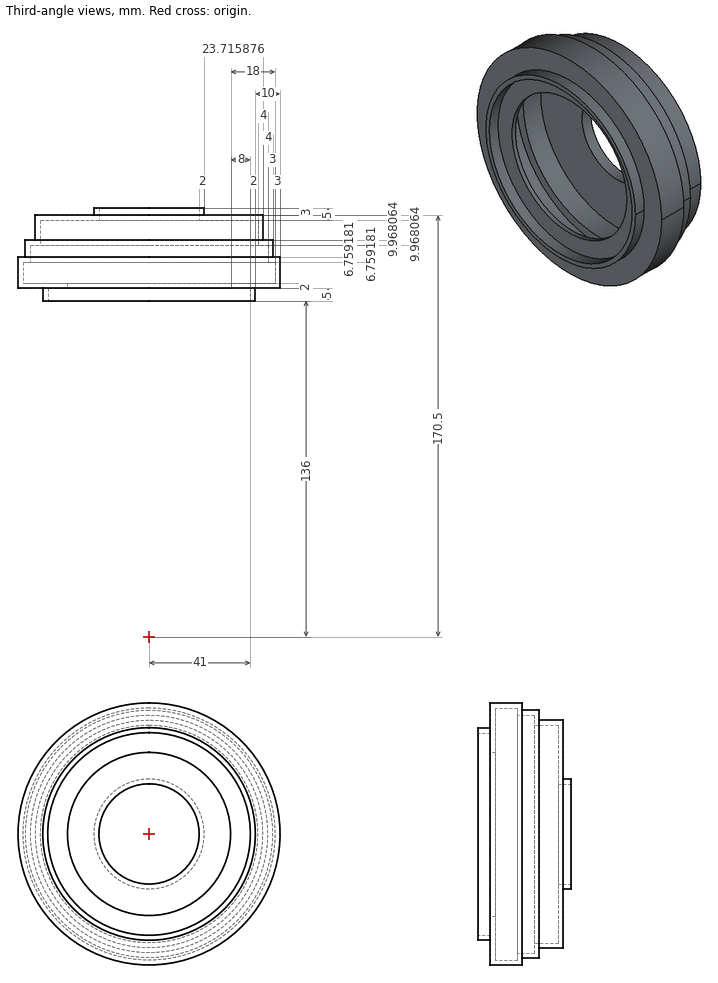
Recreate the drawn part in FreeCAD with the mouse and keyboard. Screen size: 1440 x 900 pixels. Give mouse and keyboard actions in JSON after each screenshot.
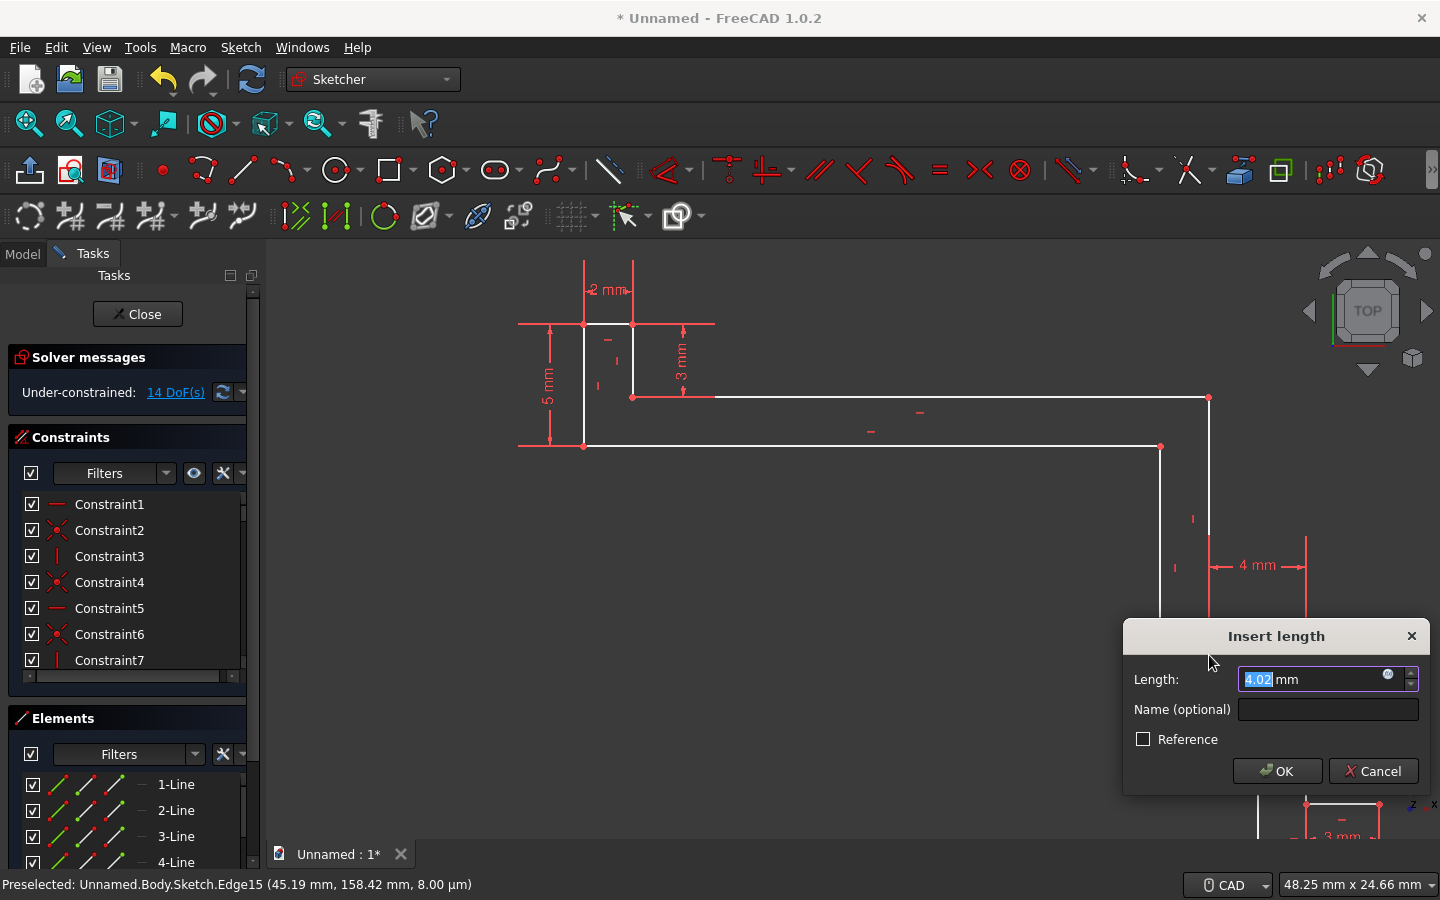
{"action": "type", "text": "4"}
{"action": "key", "text": "Return"}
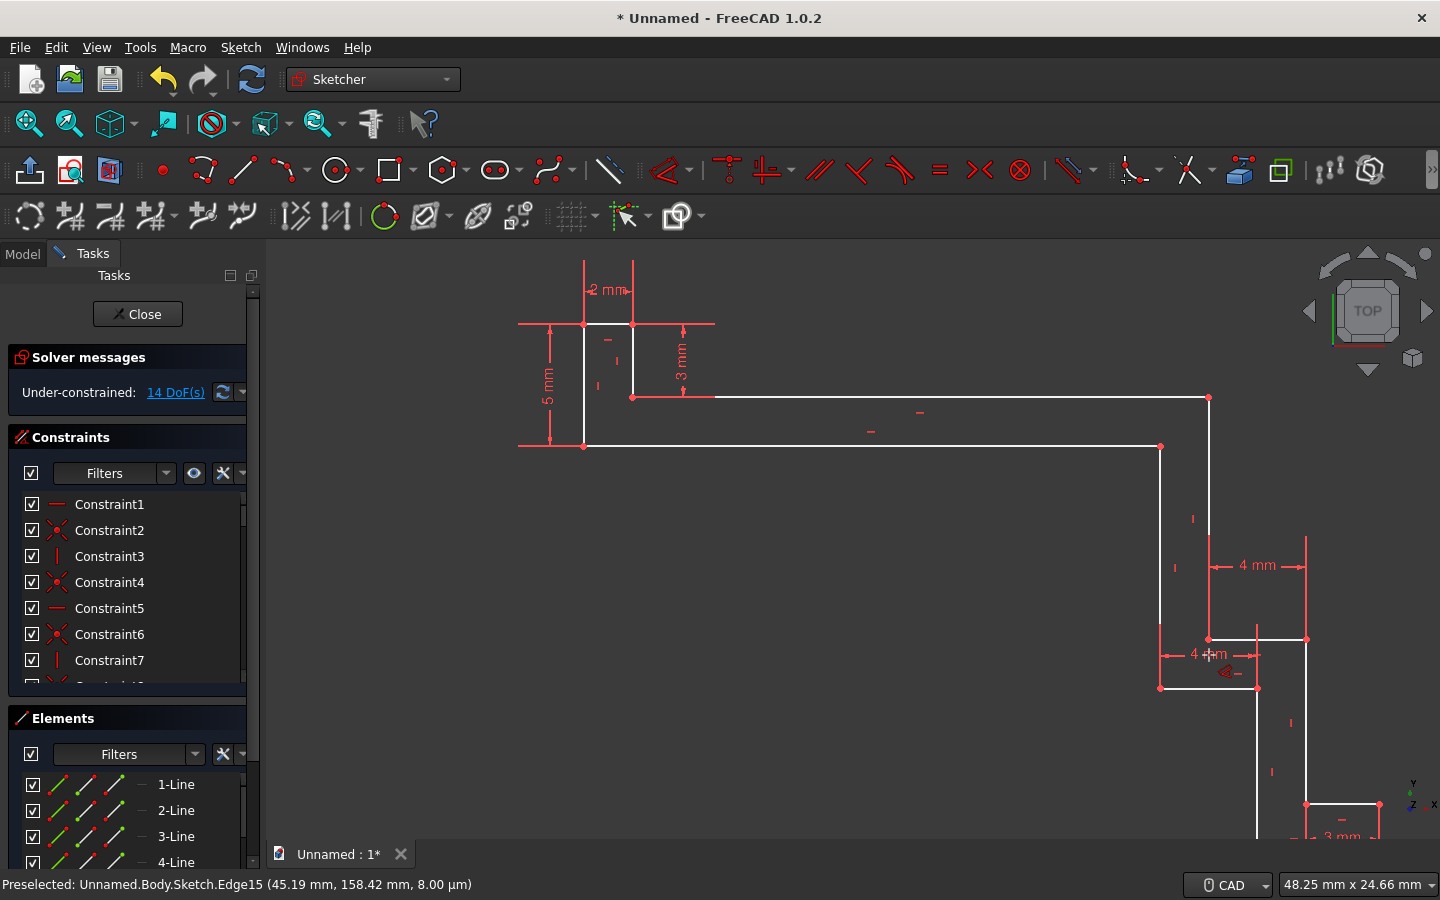
{"action": "scroll", "coordinate": [624, 344], "scroll_direction": "down", "scroll_amount": 4}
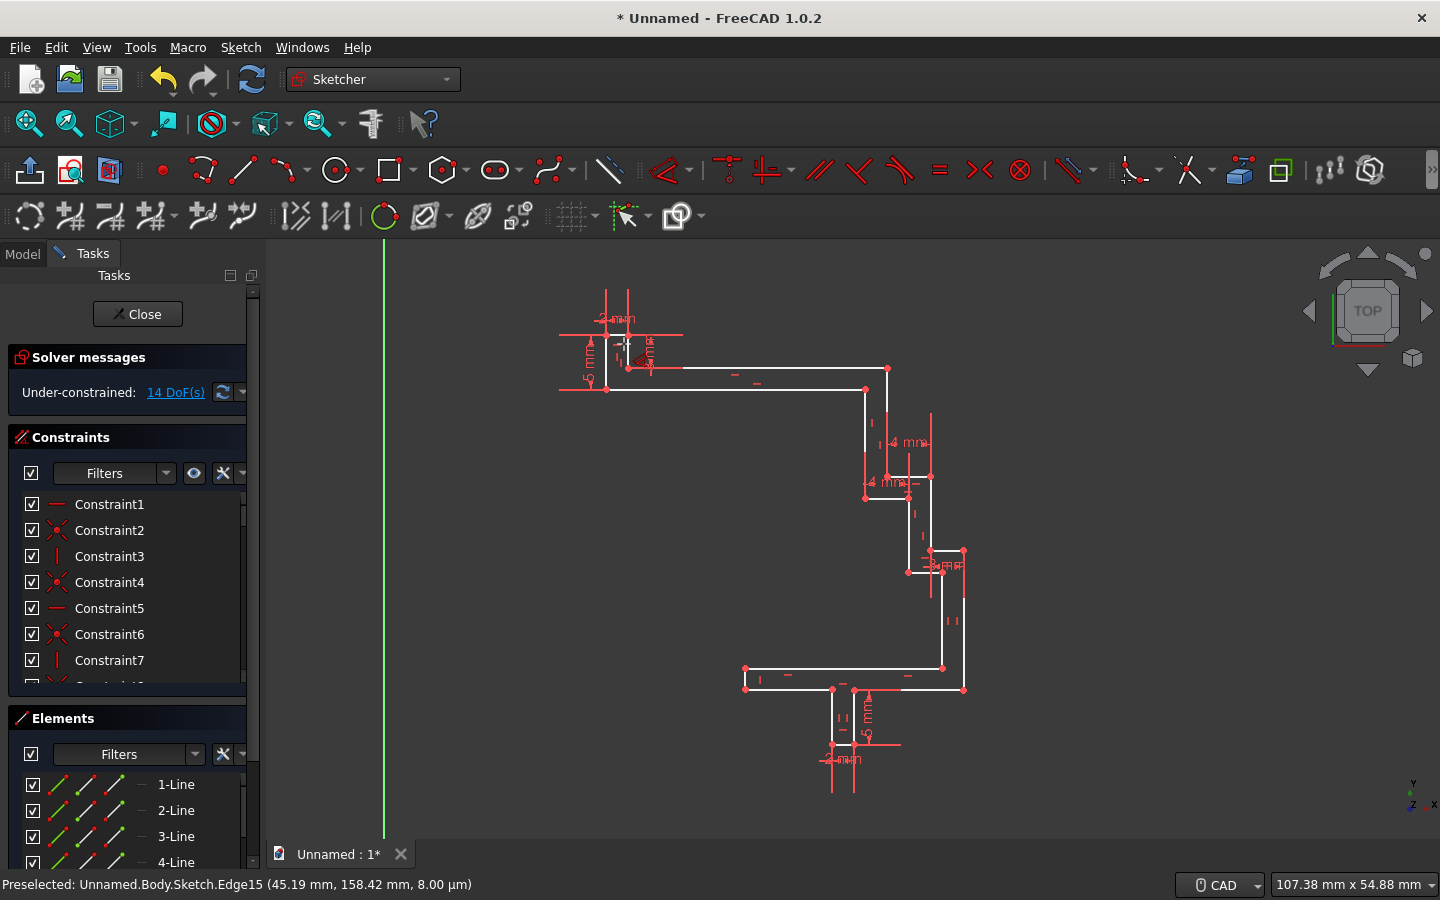
{"action": "scroll", "coordinate": [919, 573], "scroll_direction": "up", "scroll_amount": 2}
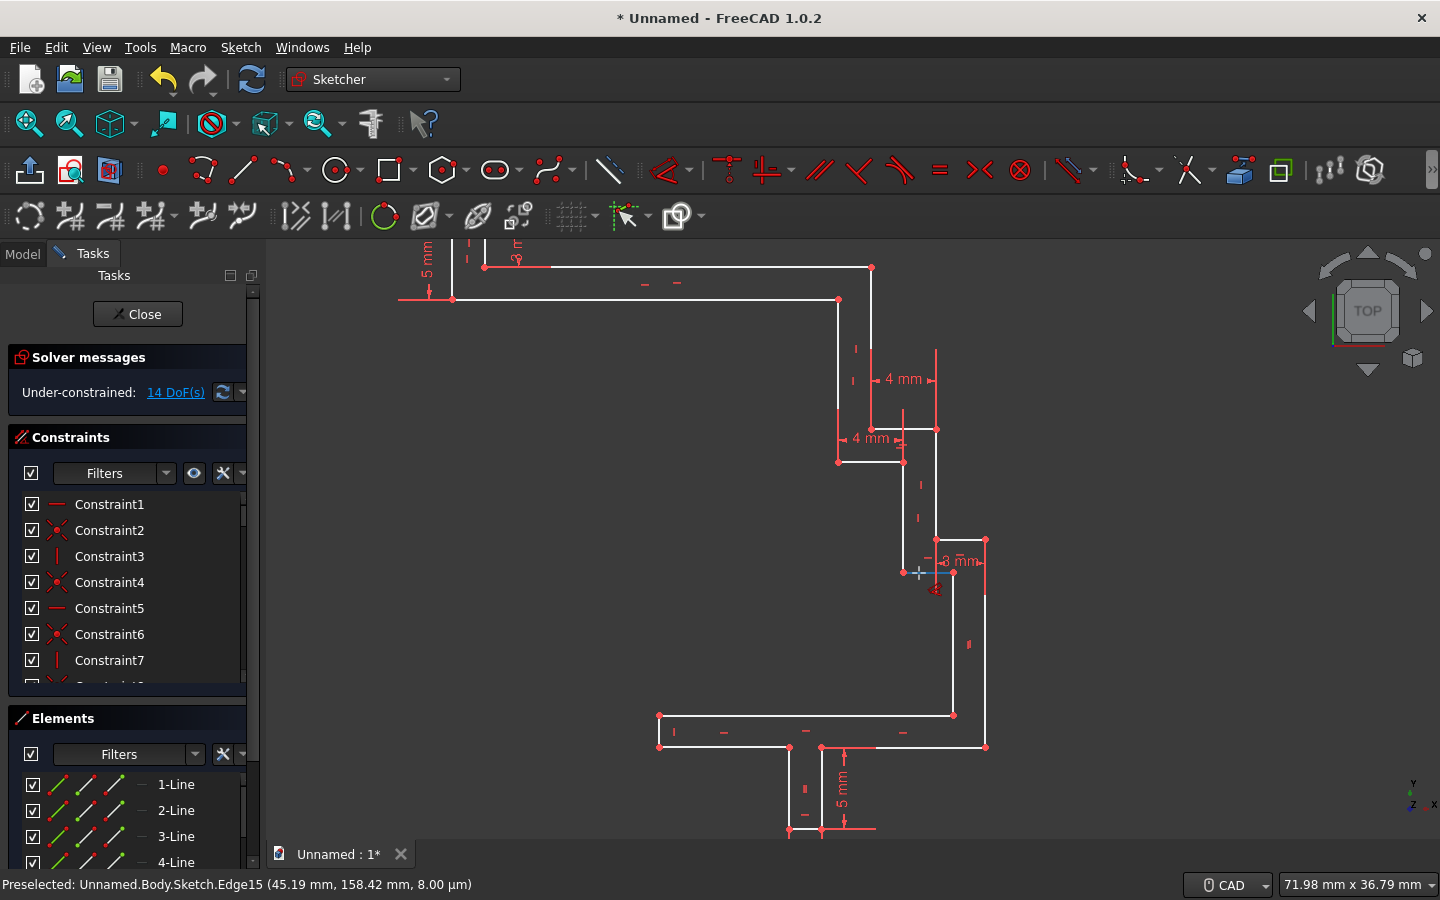
{"action": "left_click", "coordinate": [918, 573]}
{"action": "left_click", "coordinate": [928, 607]}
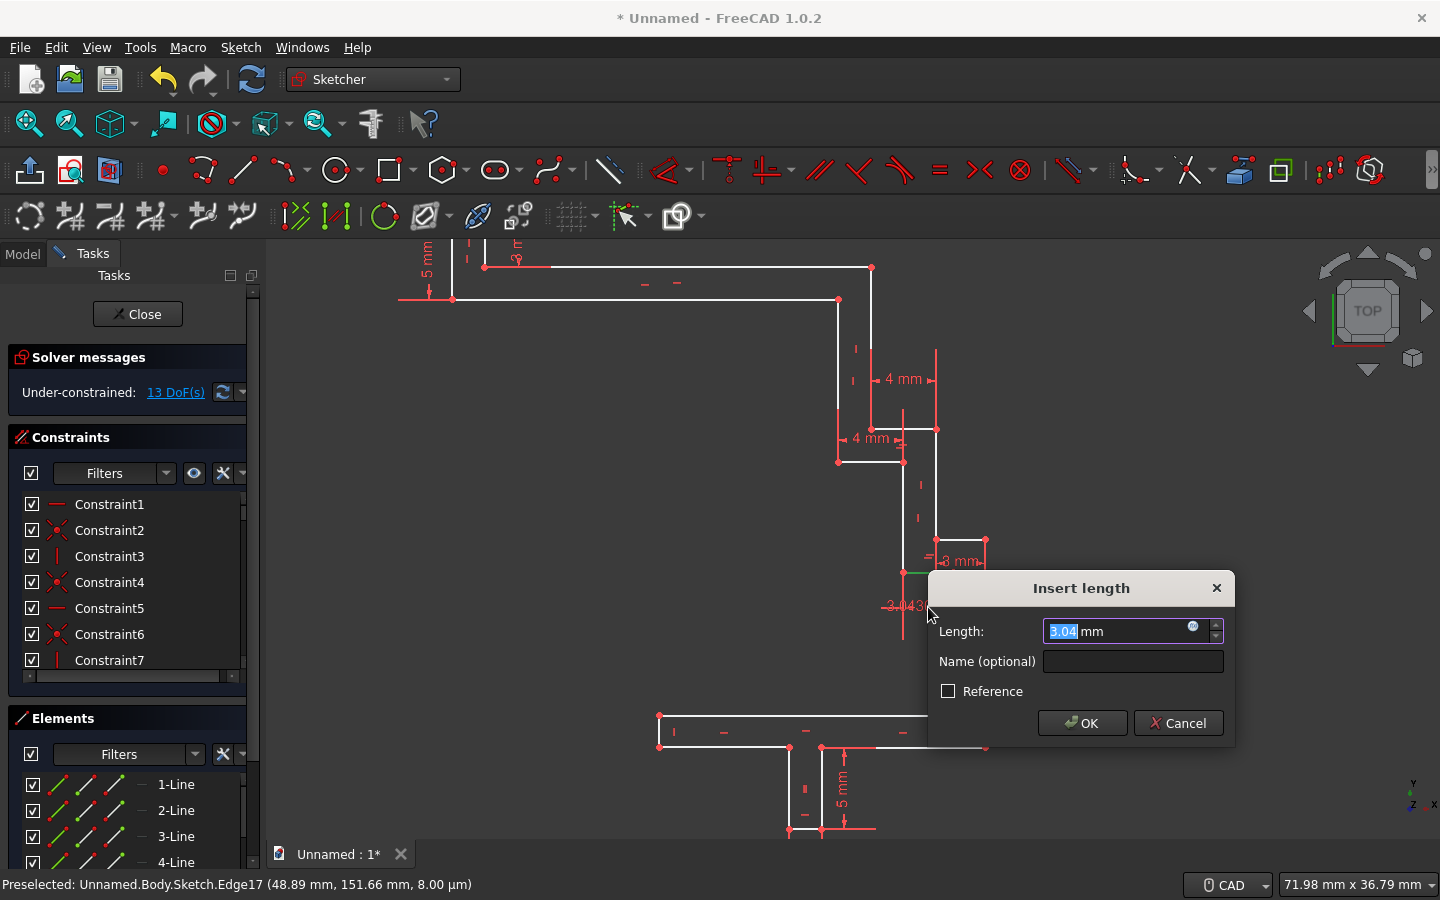
{"action": "type", "text": "3"}
{"action": "key", "text": "Return"}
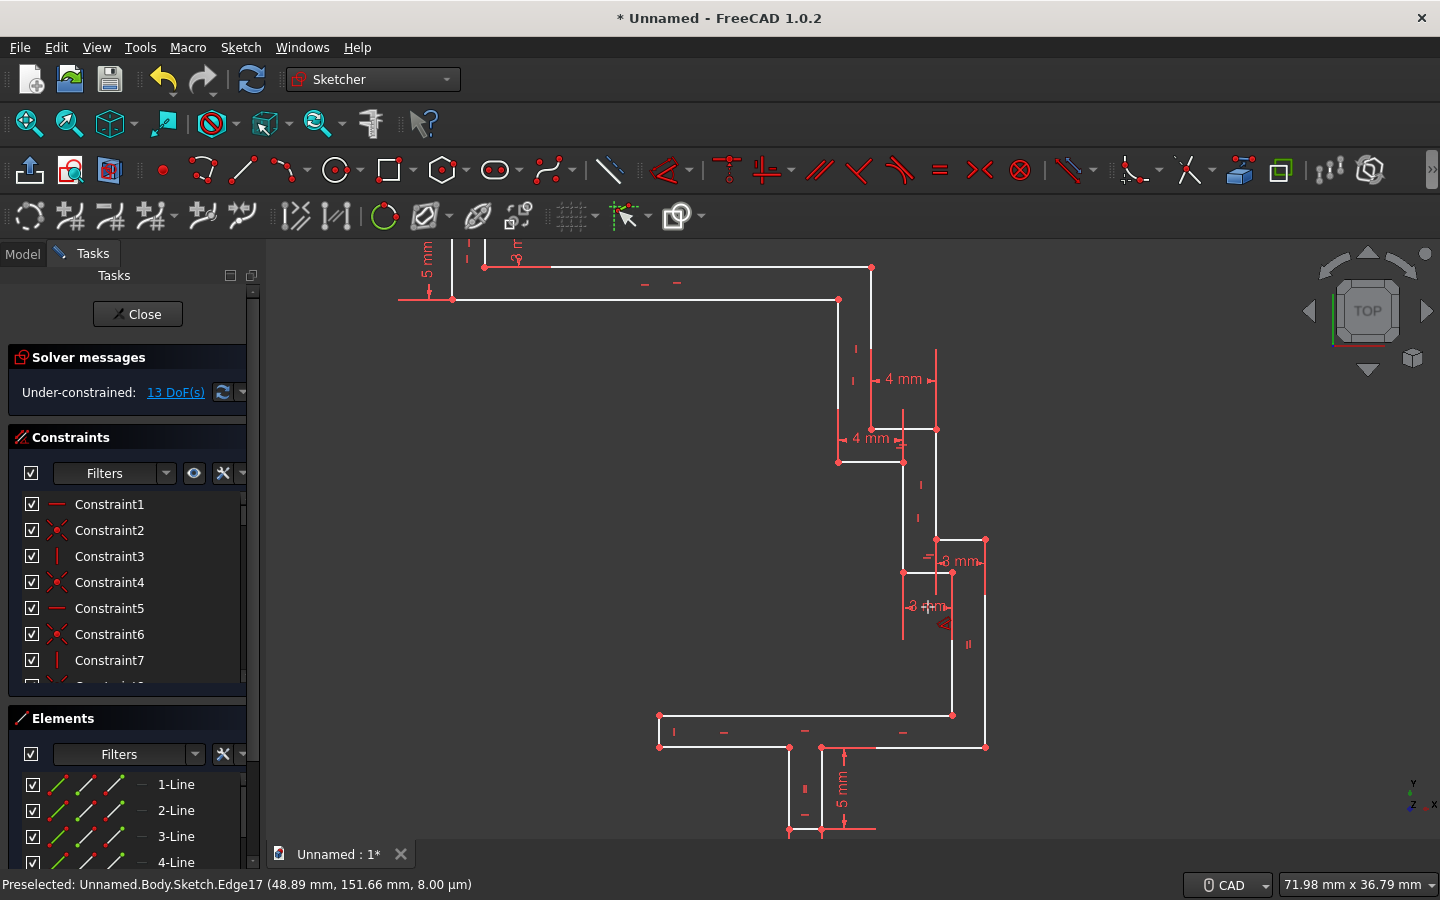
{"action": "scroll", "coordinate": [659, 725], "scroll_direction": "up", "scroll_amount": 2}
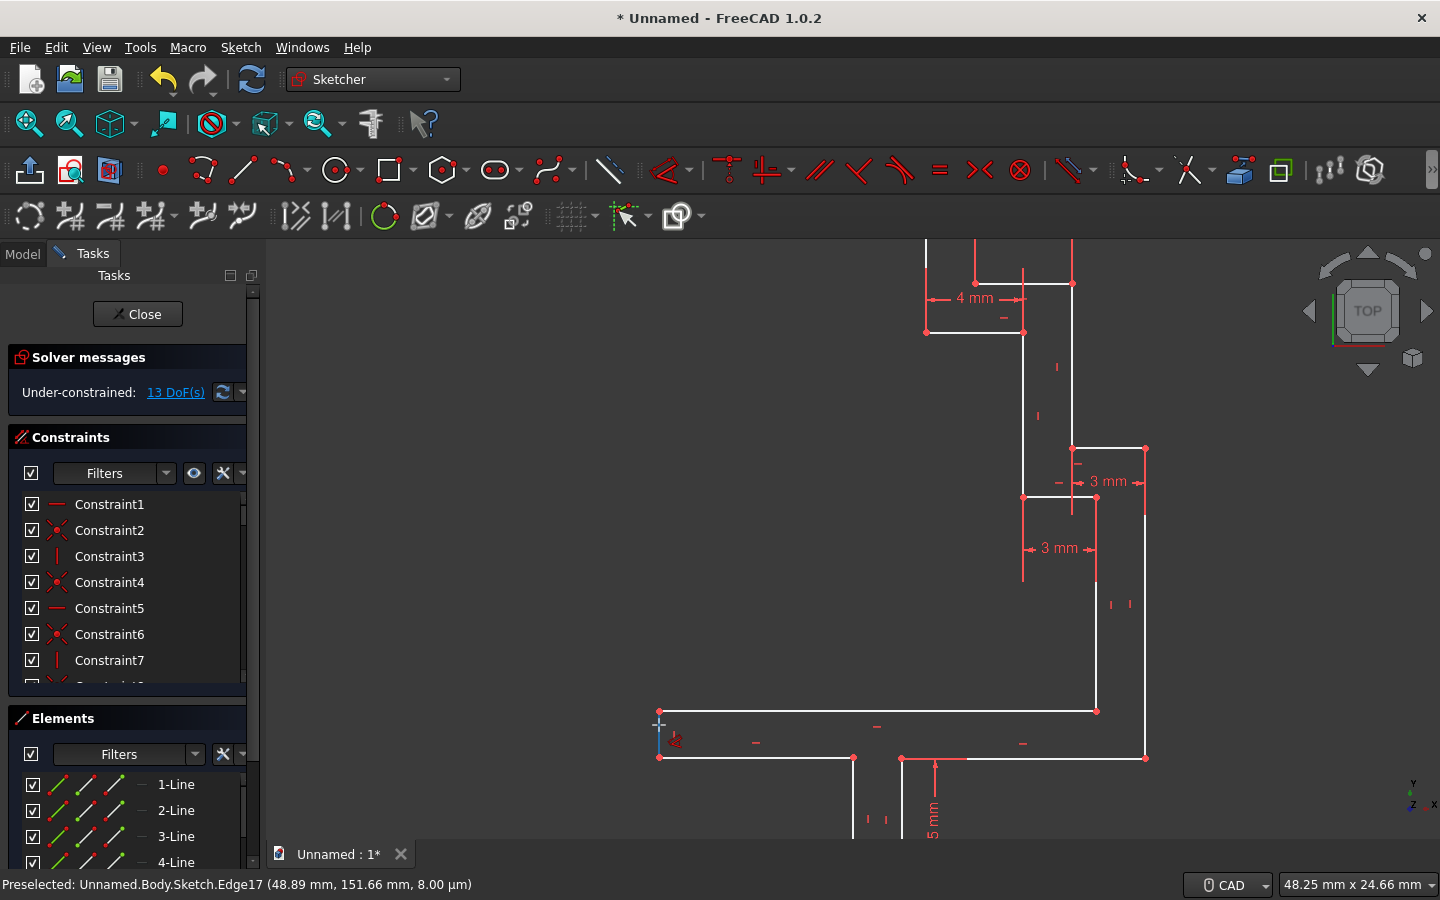
{"action": "left_click", "coordinate": [659, 725]}
{"action": "left_click", "coordinate": [625, 734]}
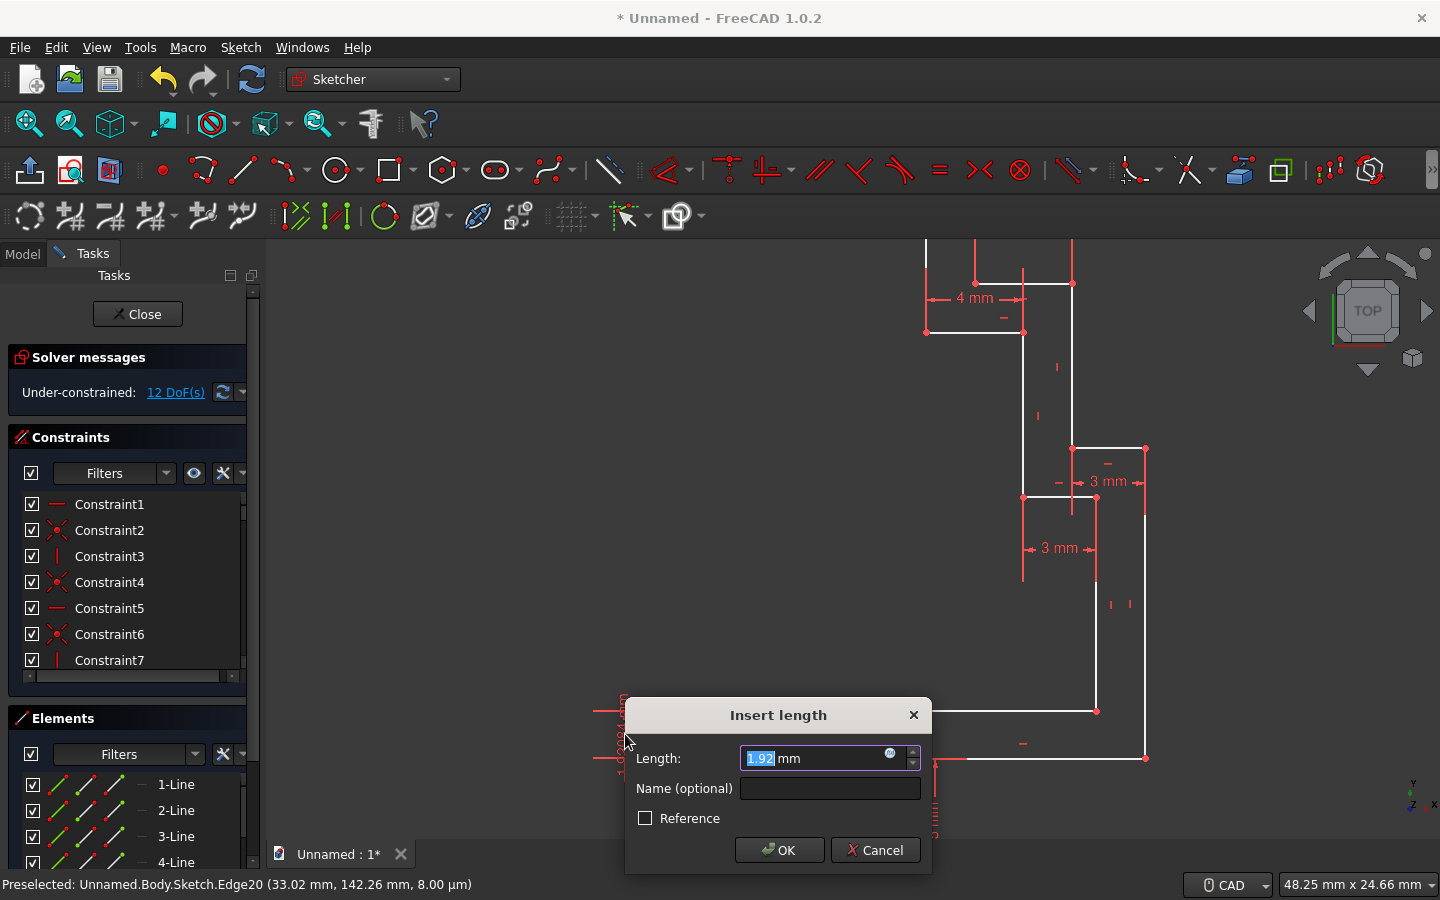
{"action": "type", "text": "2"}
{"action": "key", "text": "Return"}